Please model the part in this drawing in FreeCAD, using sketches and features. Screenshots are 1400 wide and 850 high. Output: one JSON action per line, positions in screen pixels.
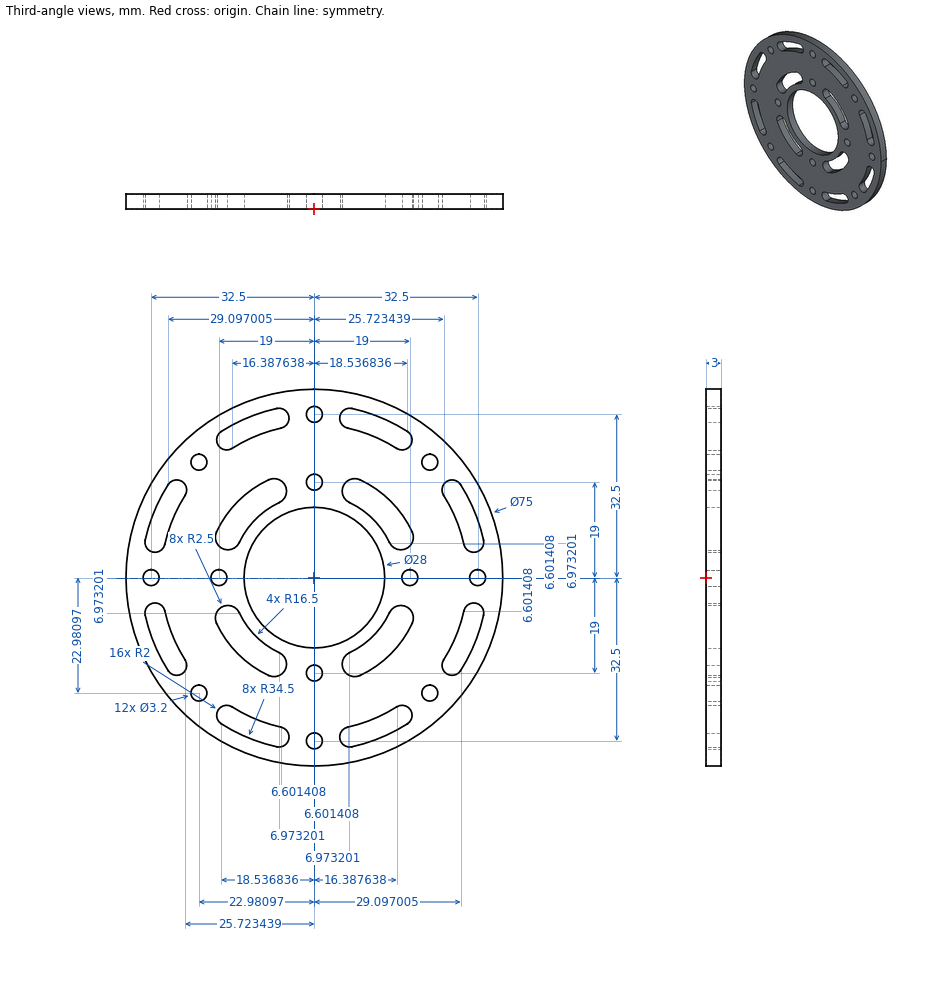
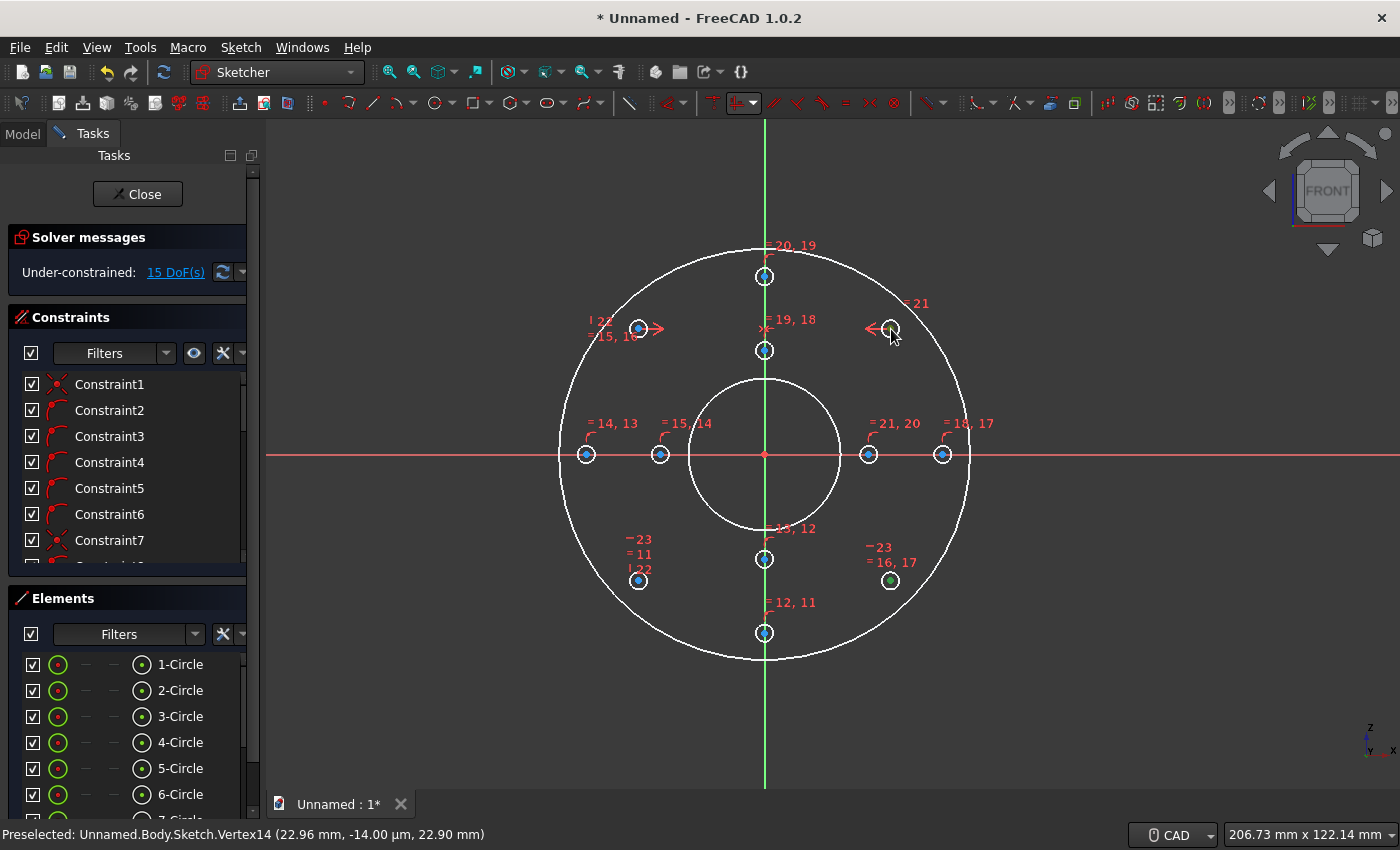
{"action": "left_click", "coordinate": [361, 455]}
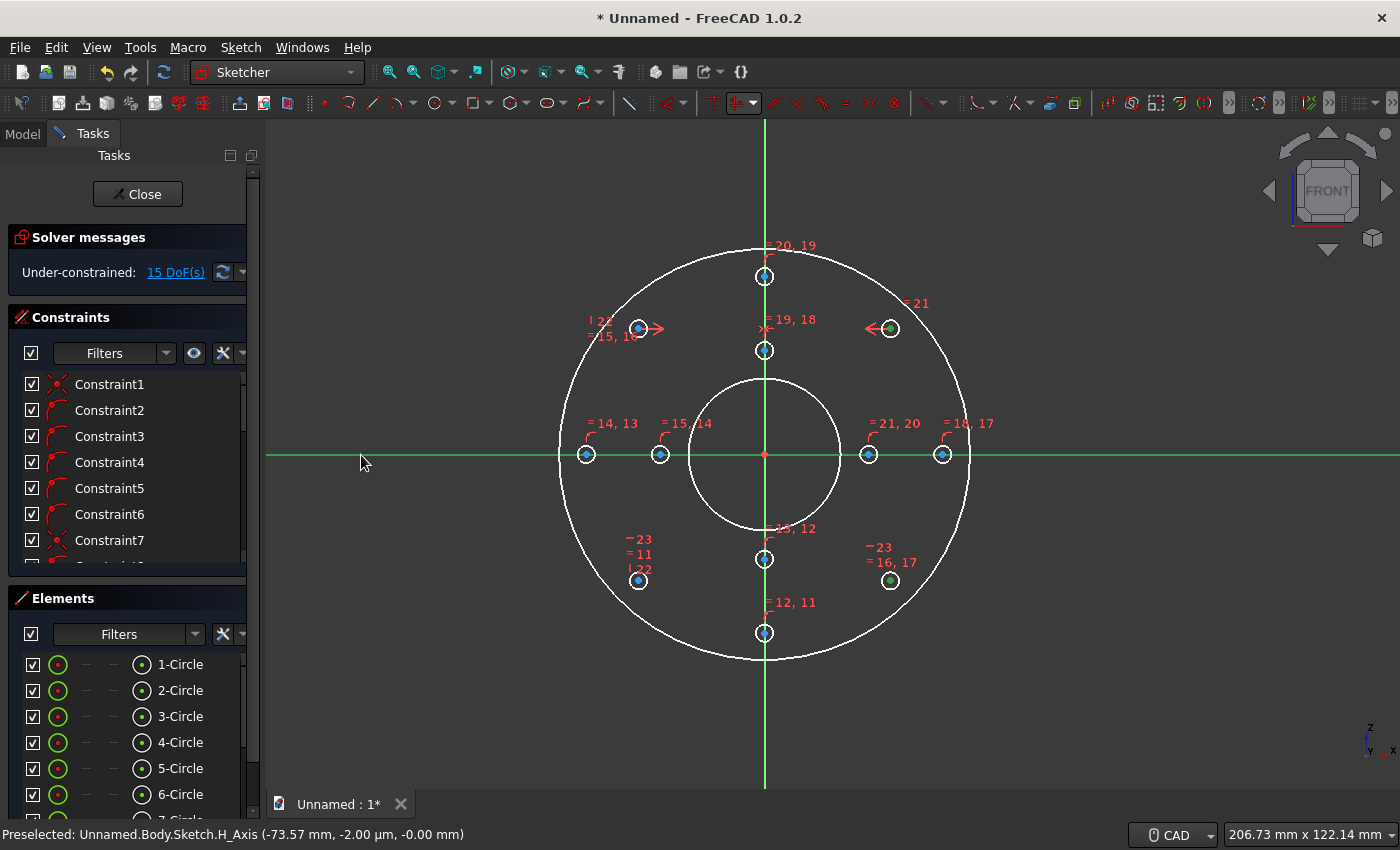
{"action": "left_click", "coordinate": [870, 104]}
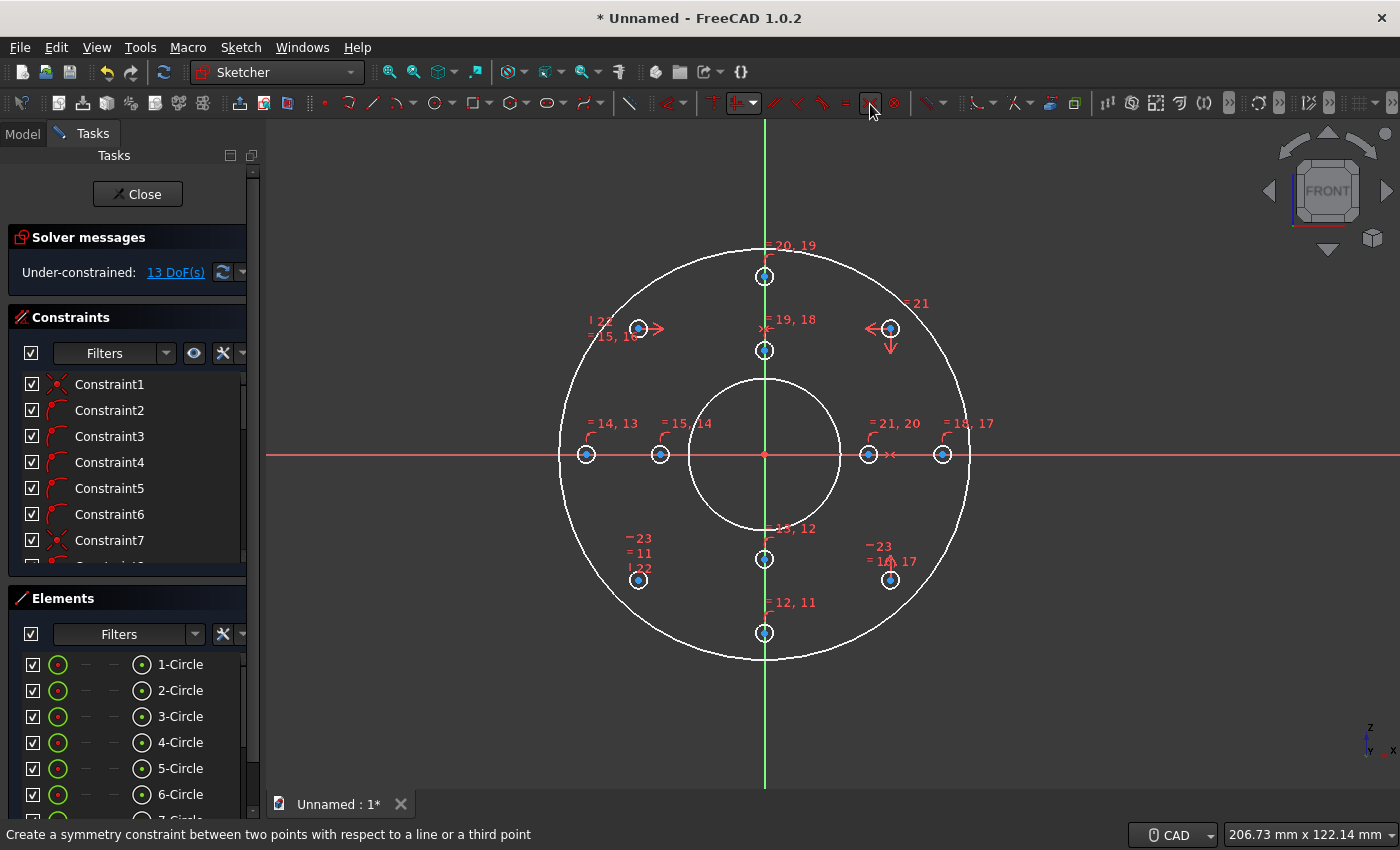
{"action": "left_click", "coordinate": [668, 104]}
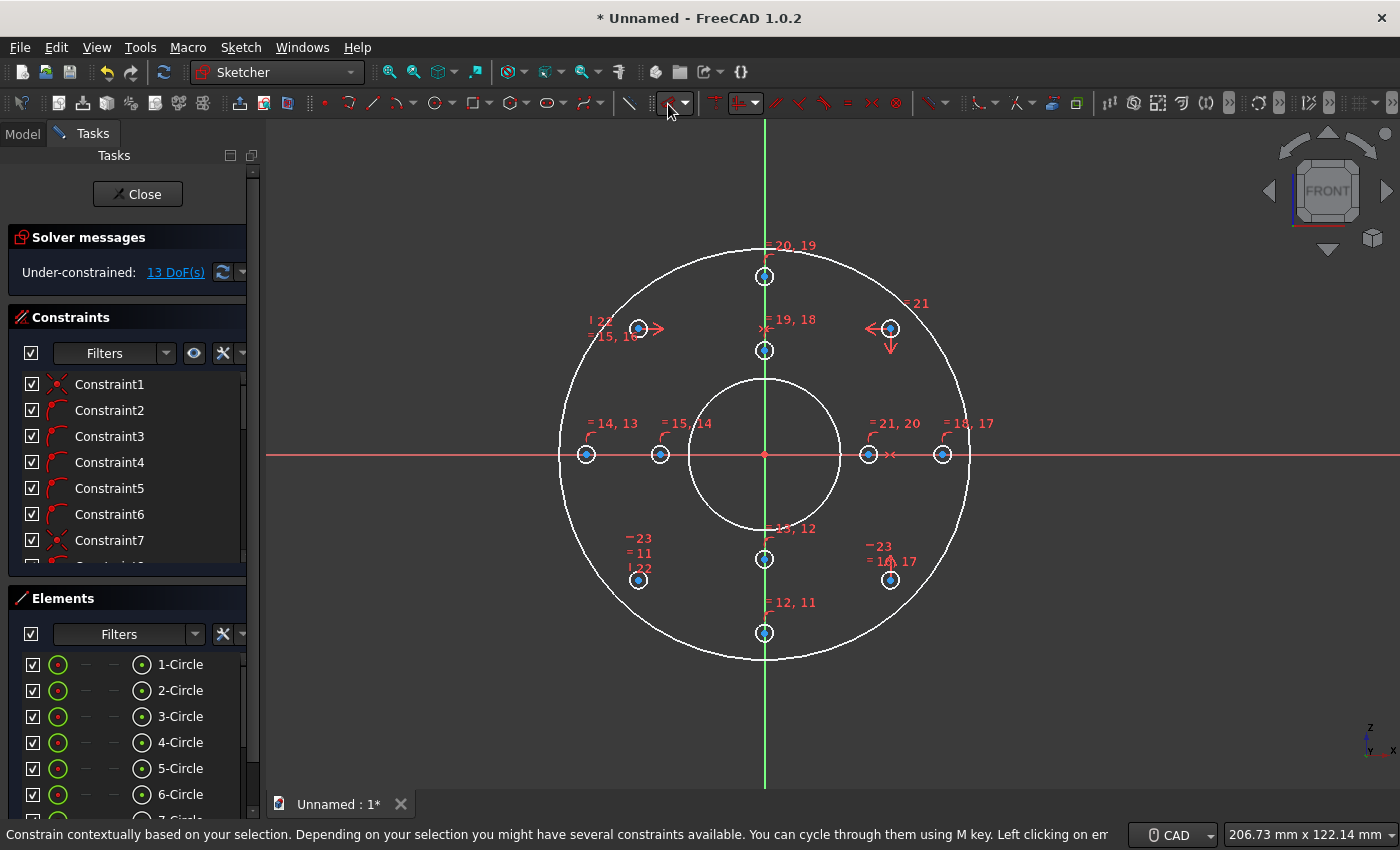
{"action": "left_click", "coordinate": [909, 309]}
{"action": "left_click", "coordinate": [932, 286]}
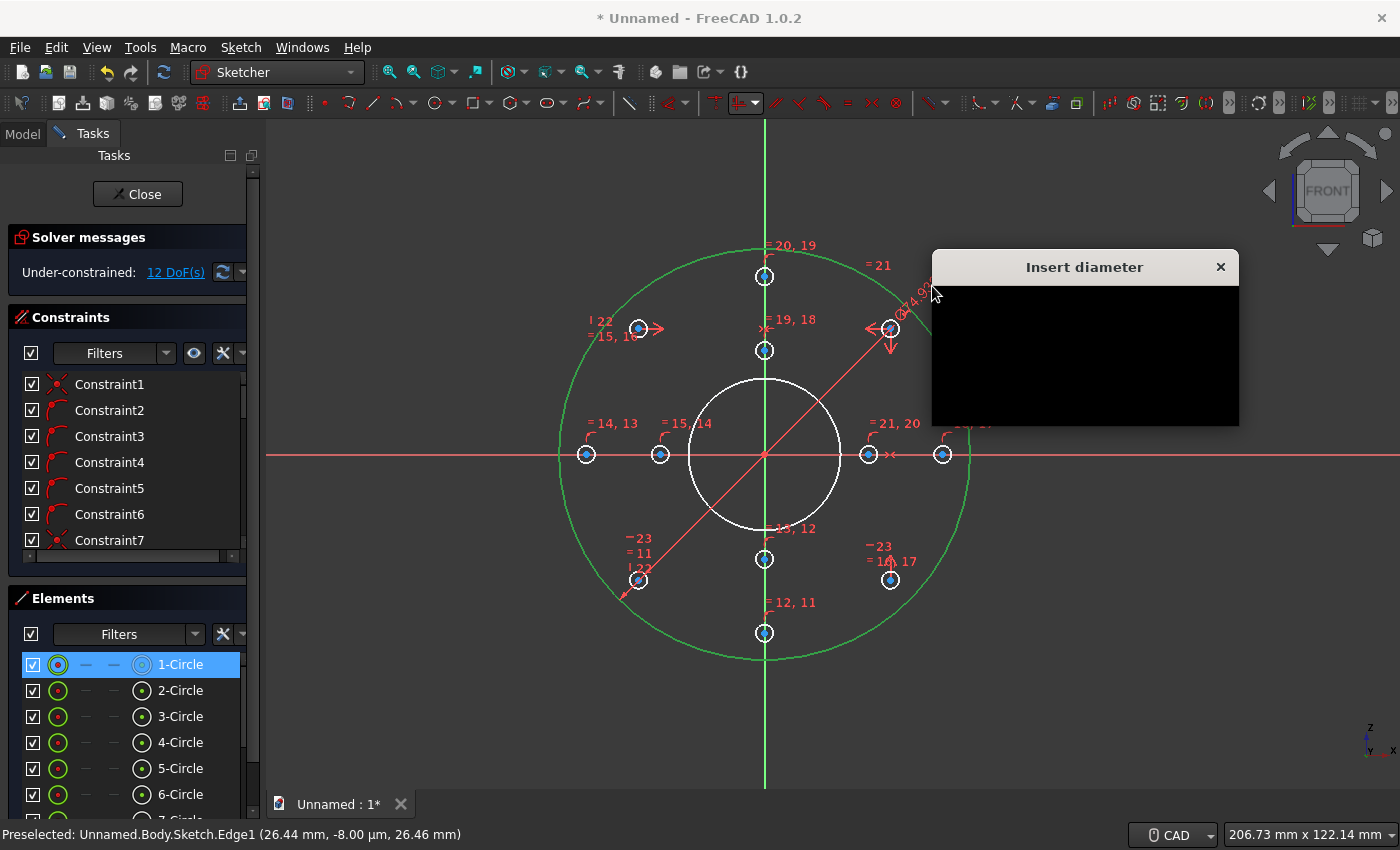
{"action": "type", "text": "75"}
{"action": "key", "text": "Return"}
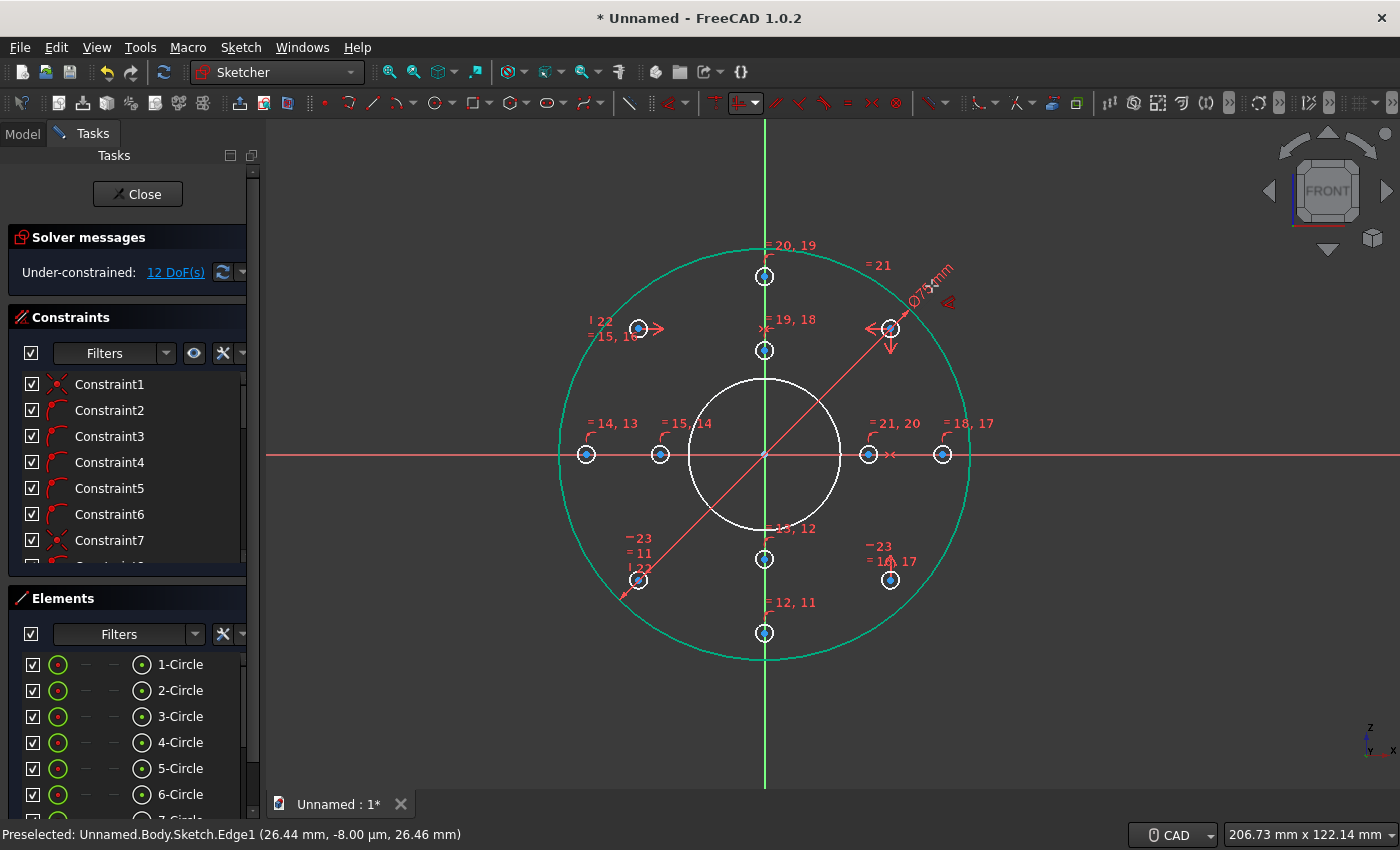
{"action": "scroll", "coordinate": [639, 572], "scroll_direction": "up", "scroll_amount": 5}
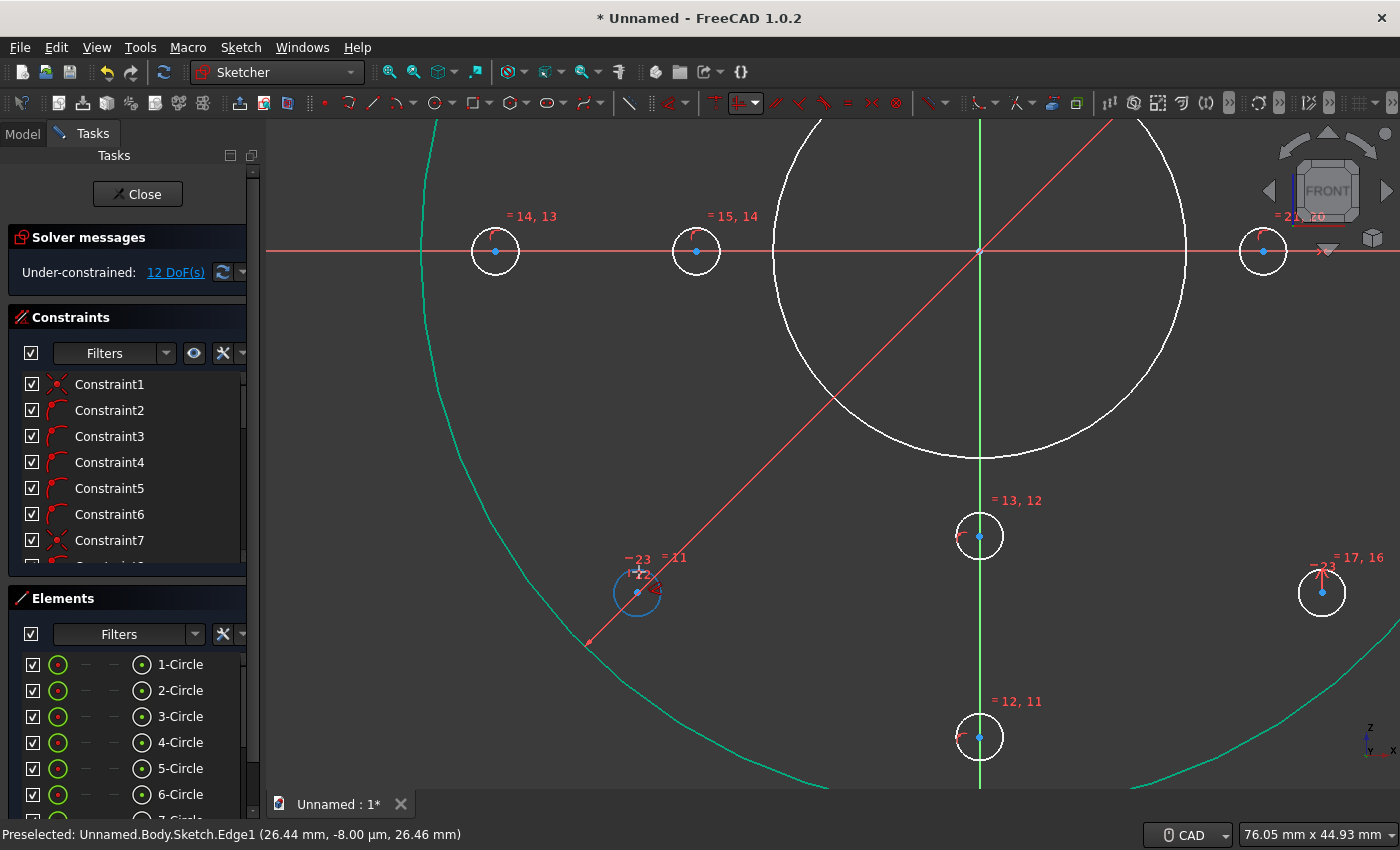
{"action": "left_click", "coordinate": [638, 570]}
{"action": "left_click", "coordinate": [639, 538]}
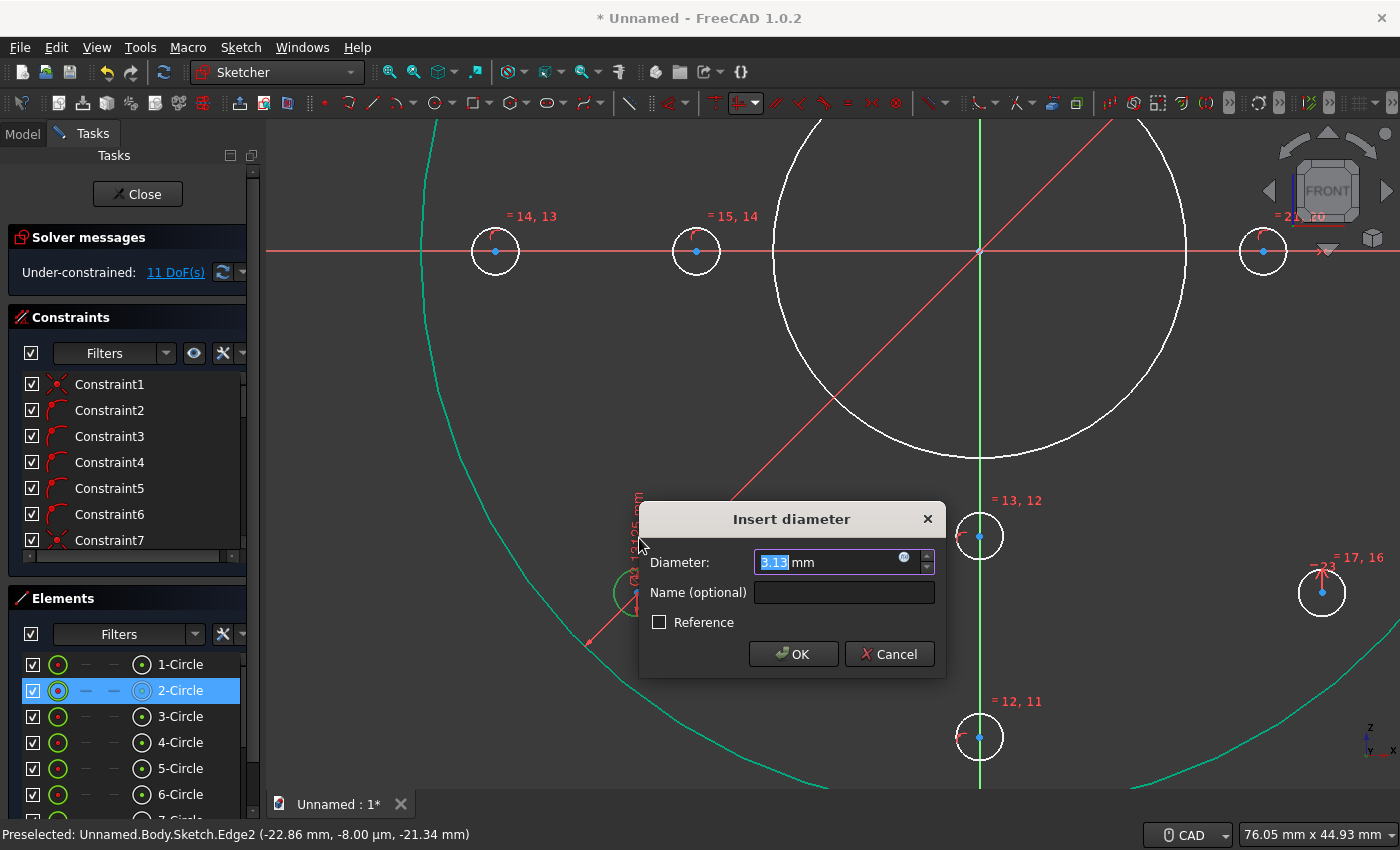
{"action": "type", "text": "3.2"}
{"action": "key", "text": "Return"}